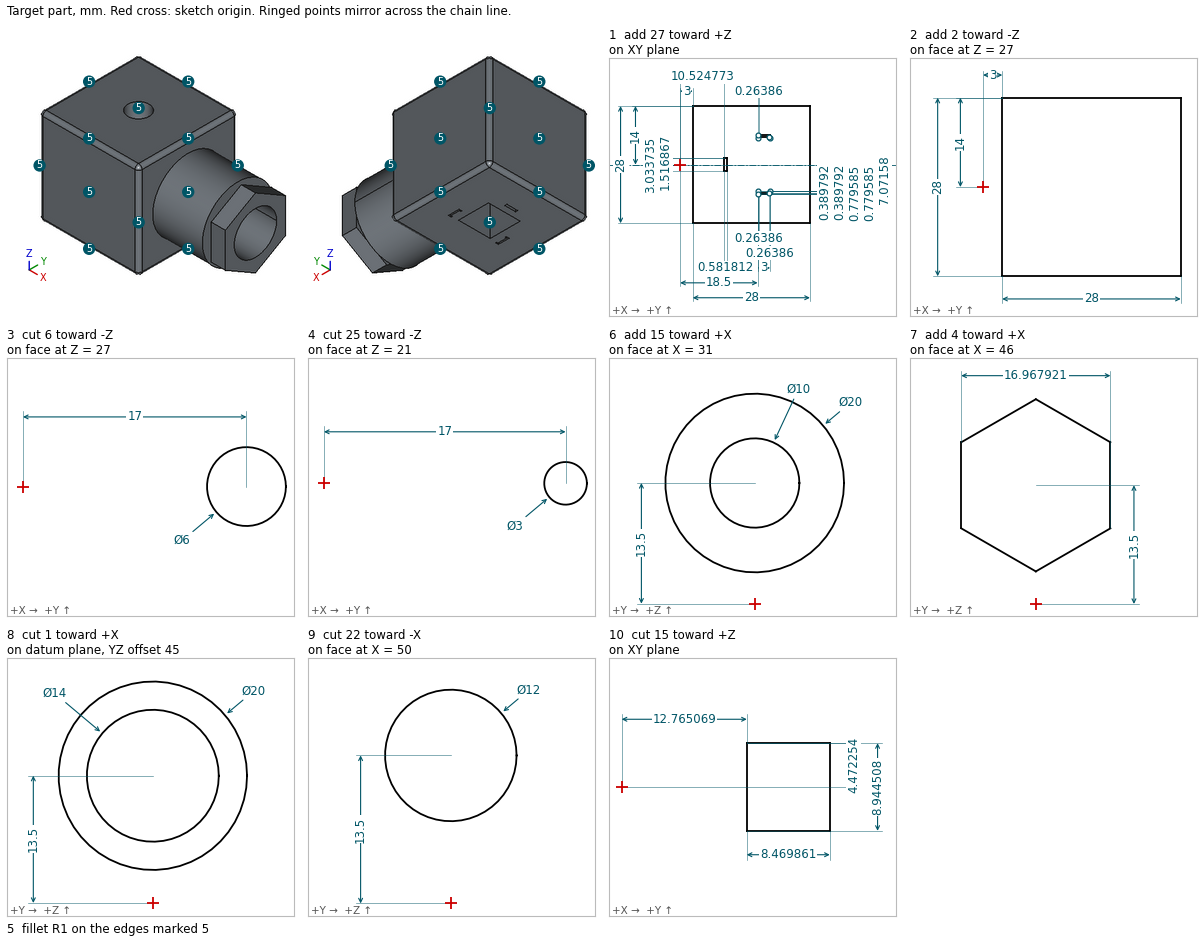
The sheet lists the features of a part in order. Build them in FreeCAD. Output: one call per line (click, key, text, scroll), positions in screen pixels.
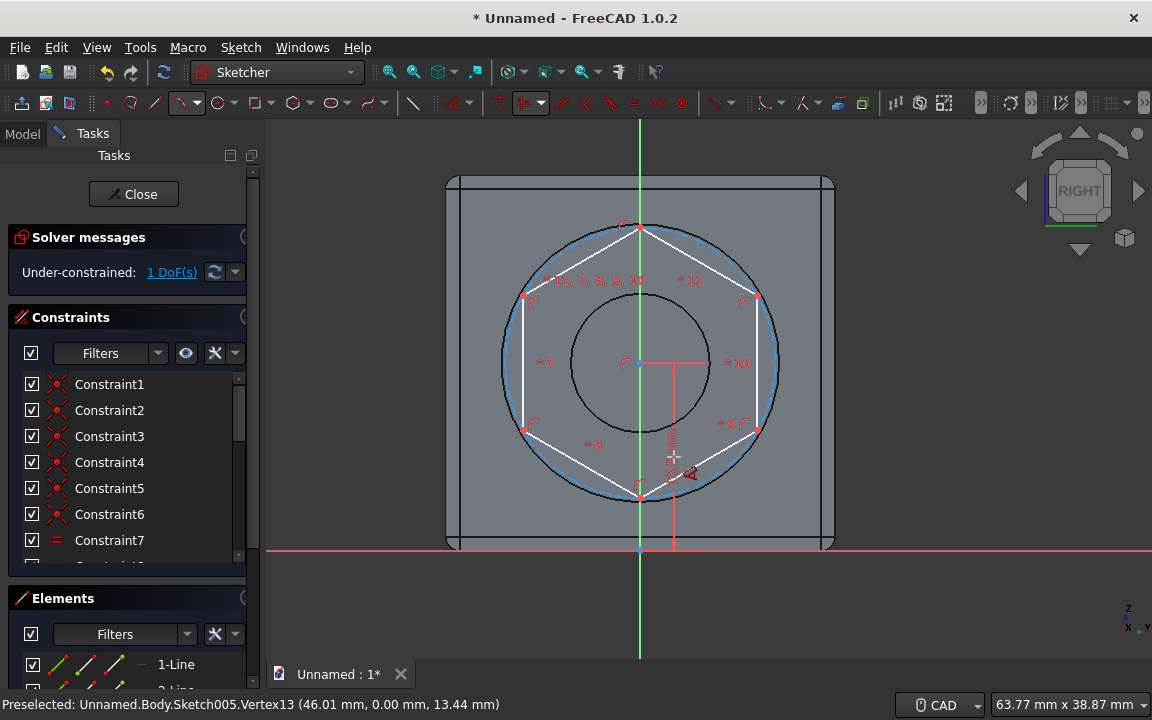
click(523, 296)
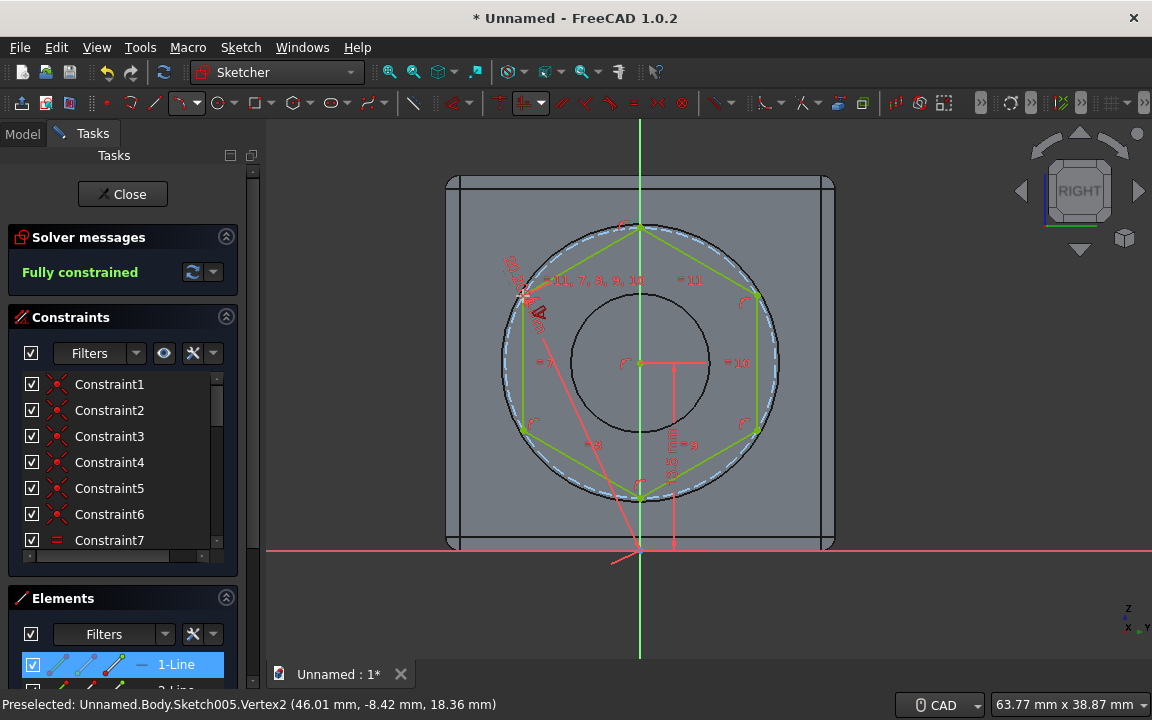
click(757, 431)
click(558, 238)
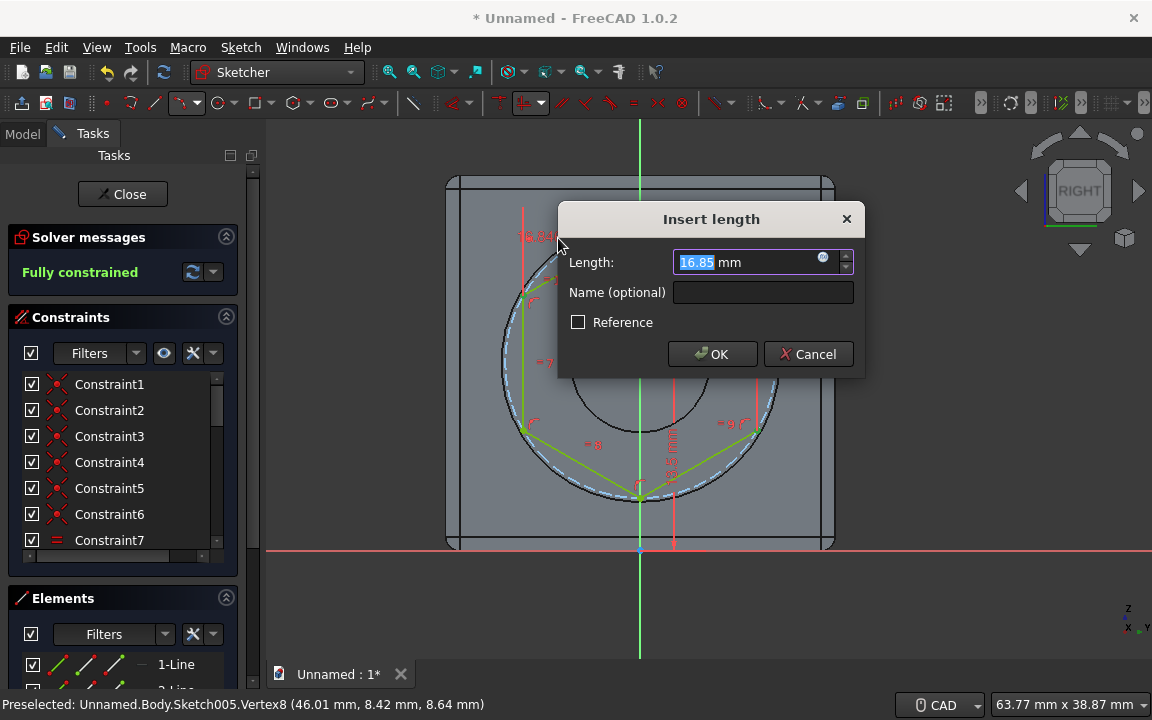
text(16.967921)
key(Return)
key(Escape)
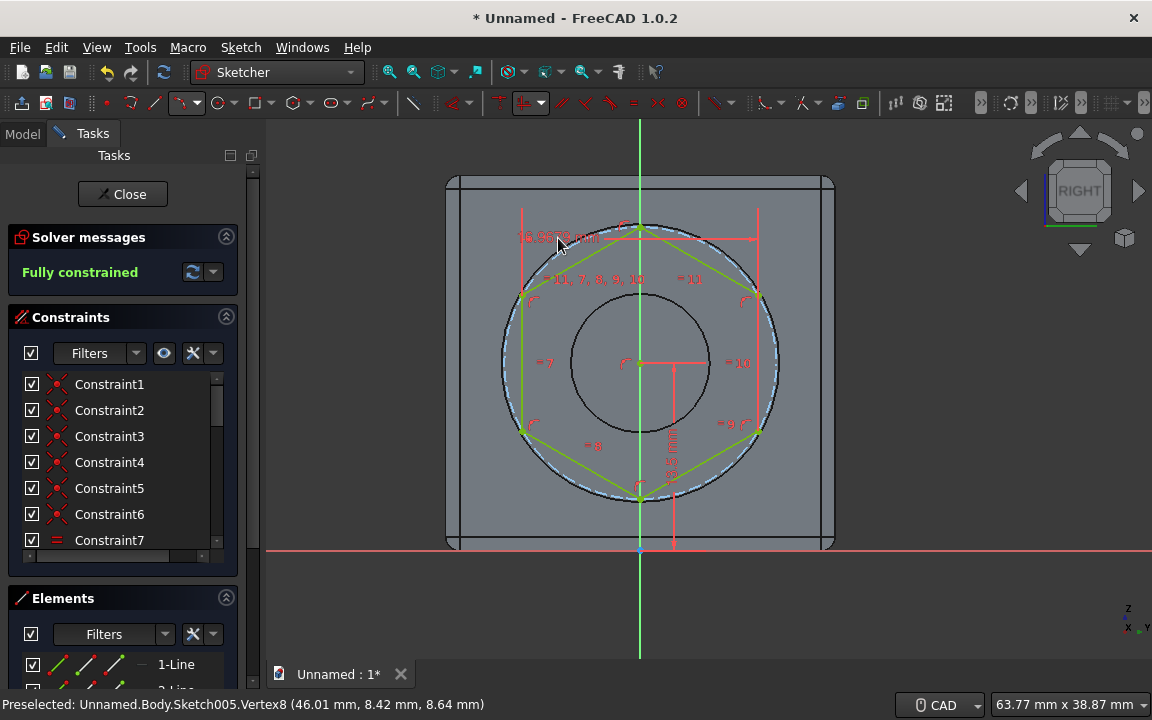
click(123, 194)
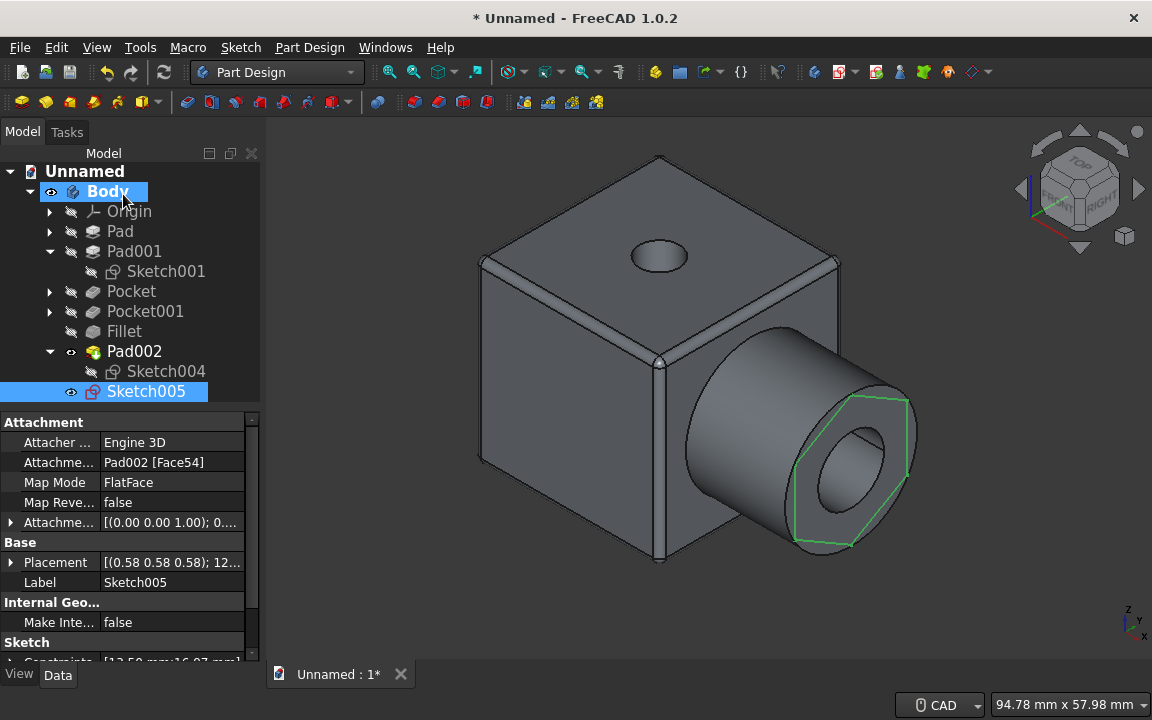
click(22, 102)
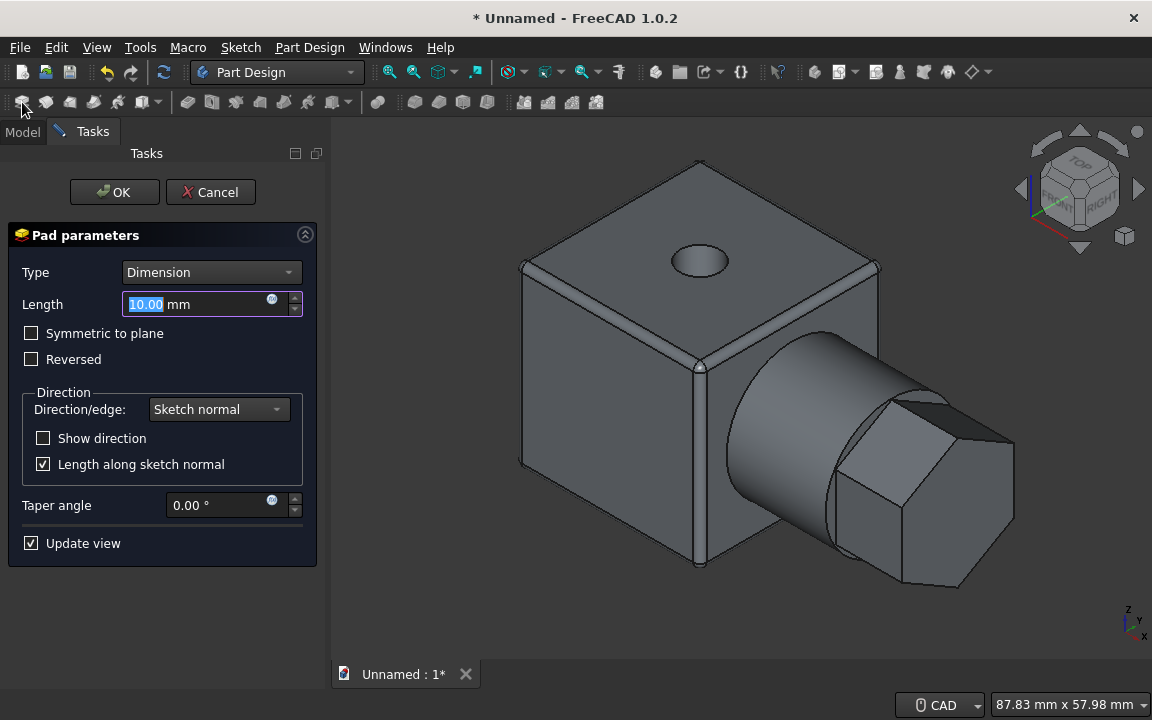
text(4)
key(Tab)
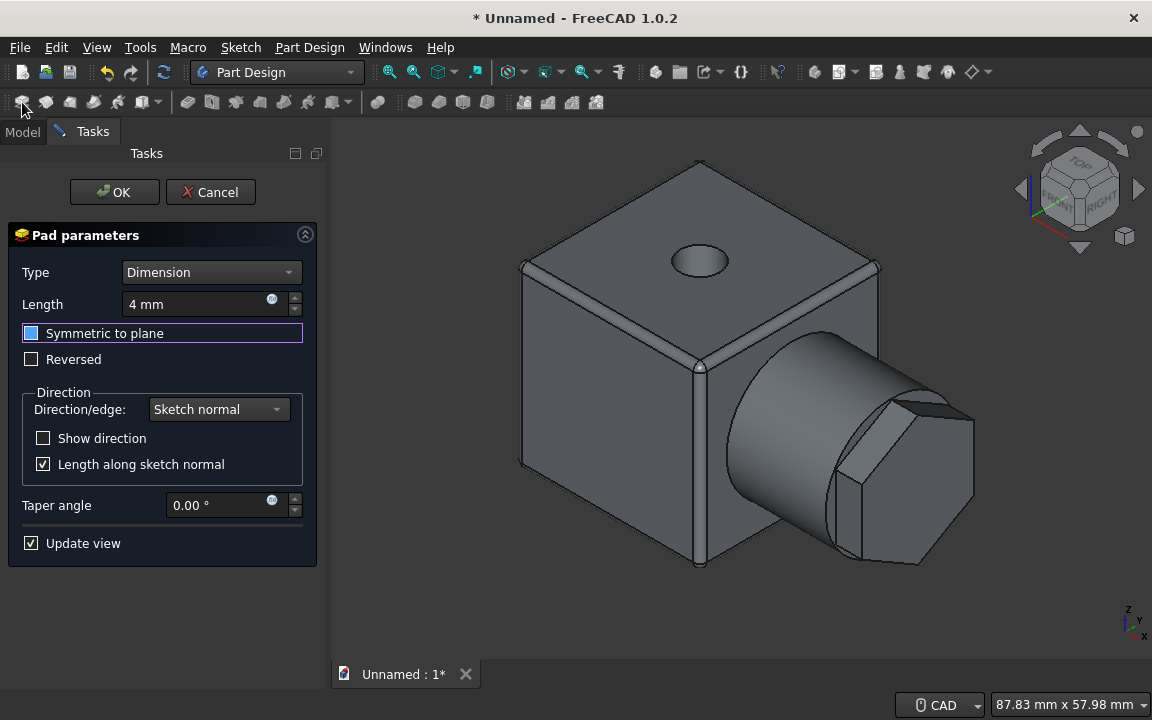
click(115, 192)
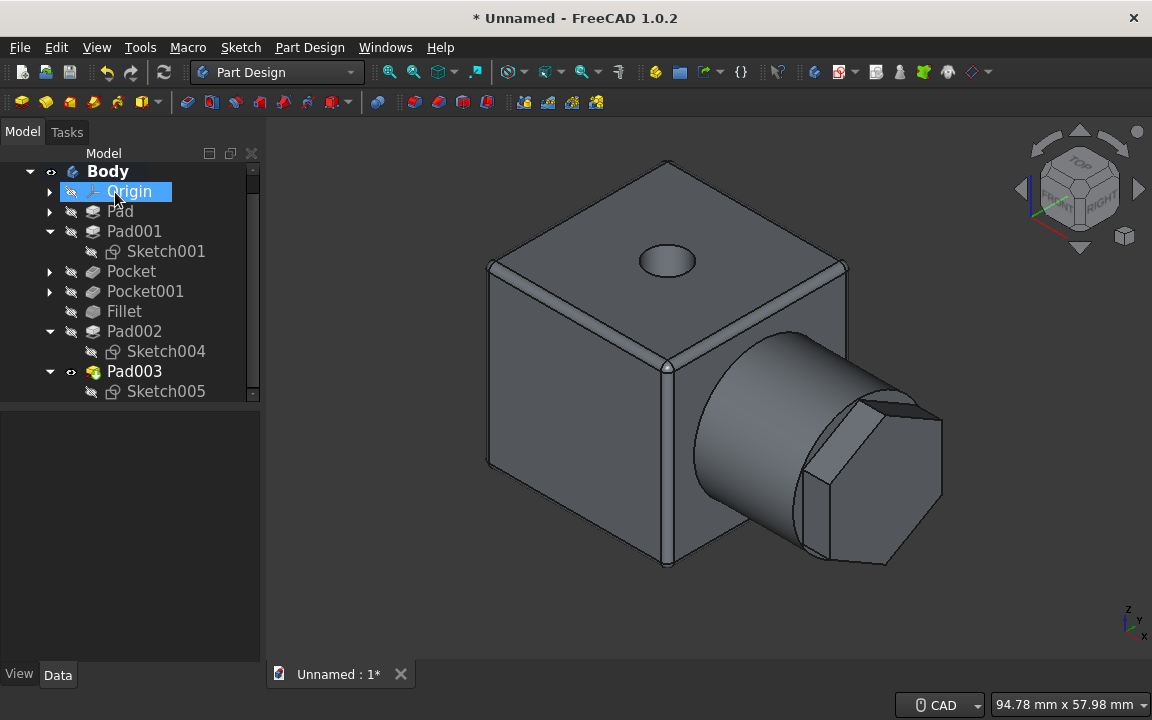
click(50, 192)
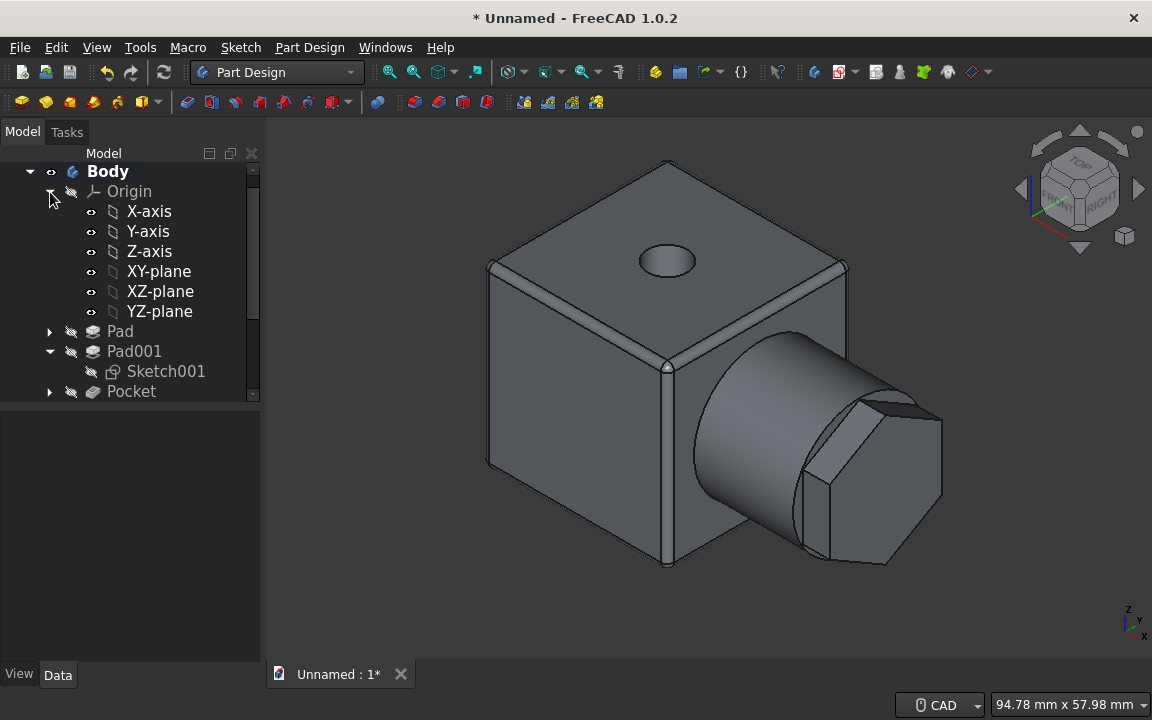
click(136, 312)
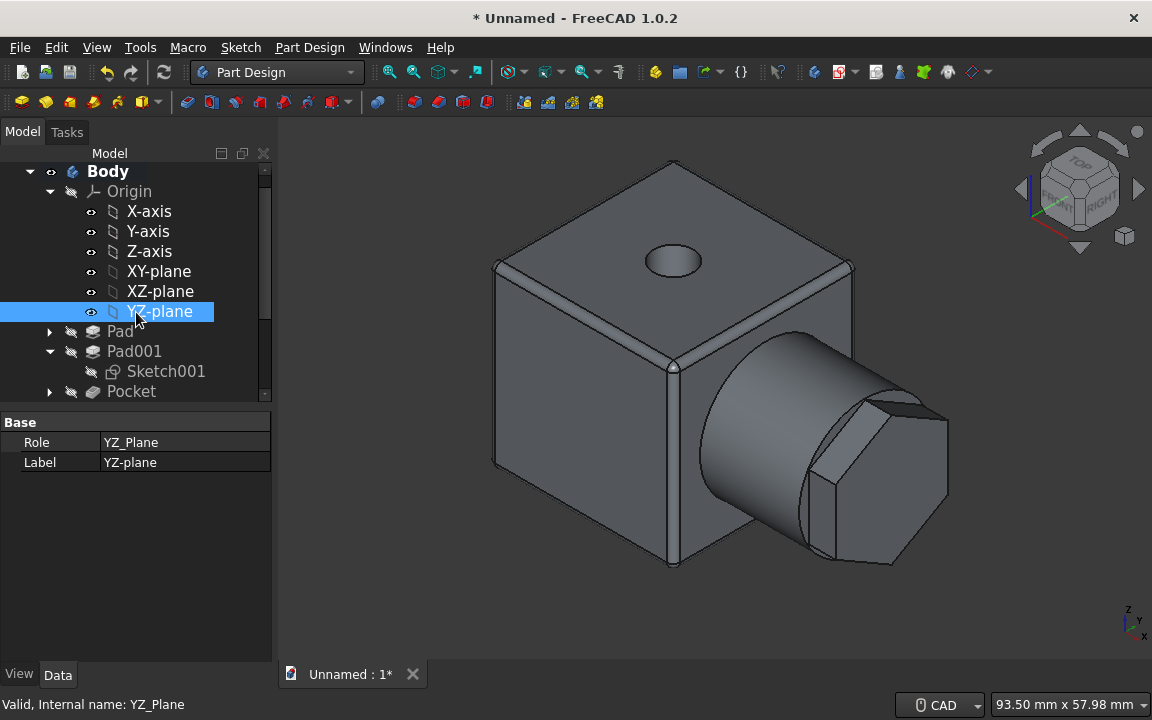
click(972, 72)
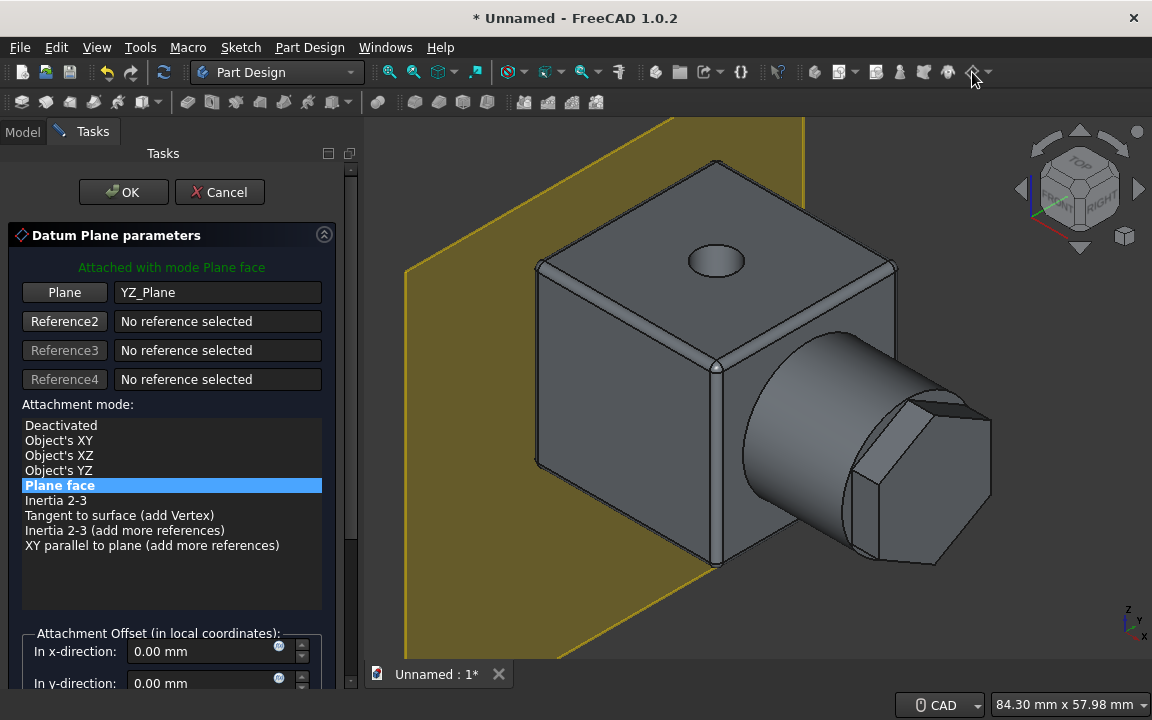
scroll(351, 426, down, 2)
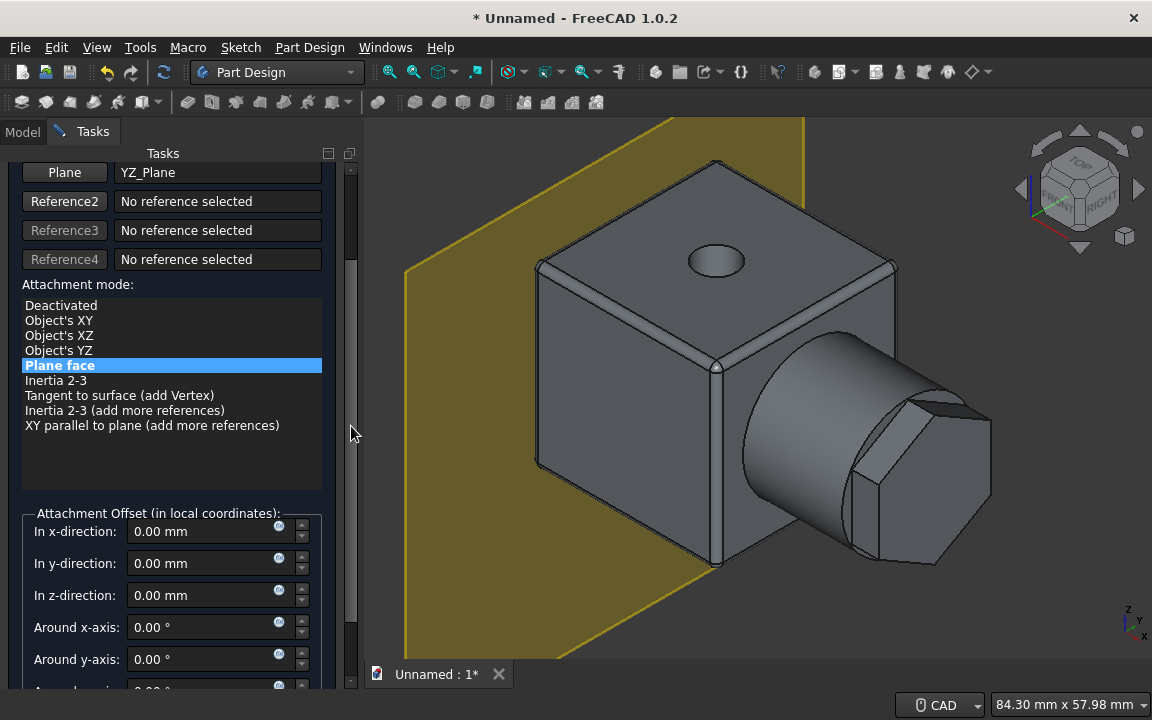
triple_click(210, 595)